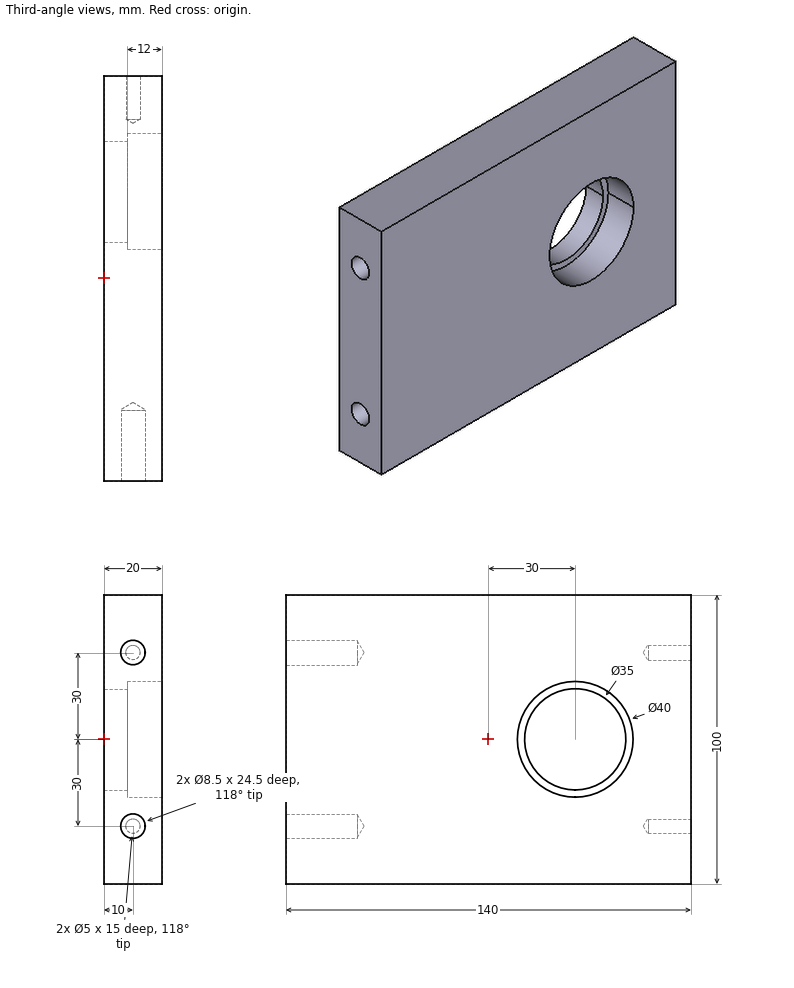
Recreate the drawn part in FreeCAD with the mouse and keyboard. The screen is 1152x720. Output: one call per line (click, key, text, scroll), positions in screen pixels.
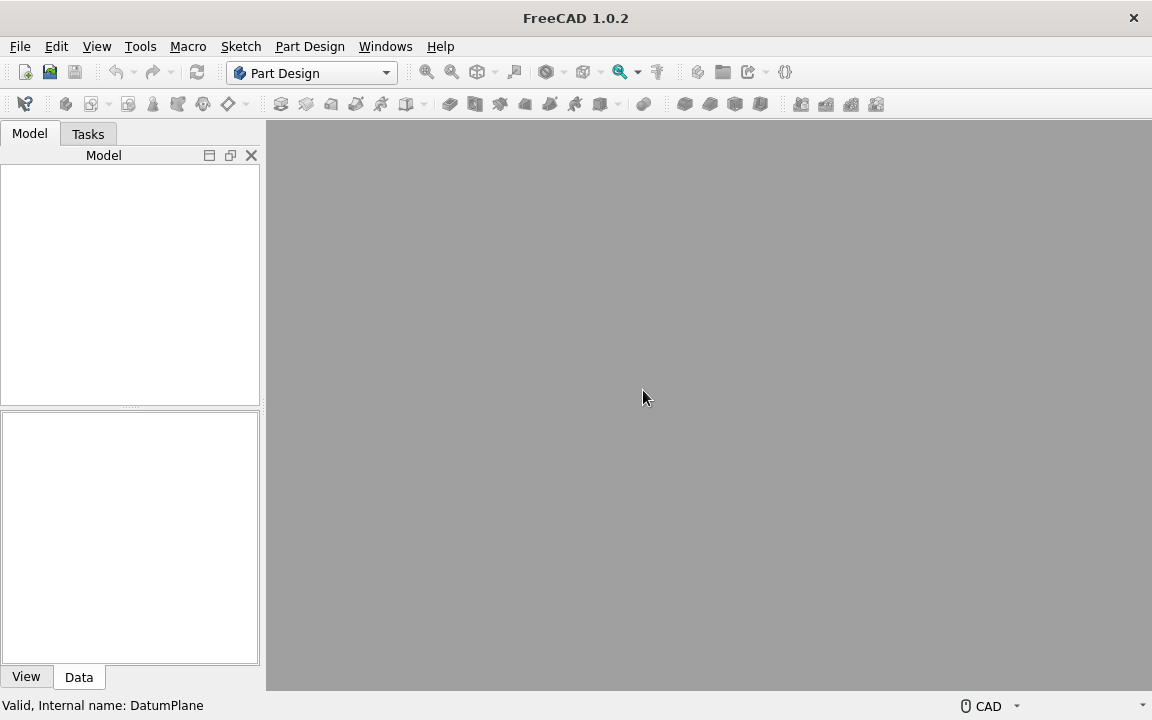
key(ctrl+n)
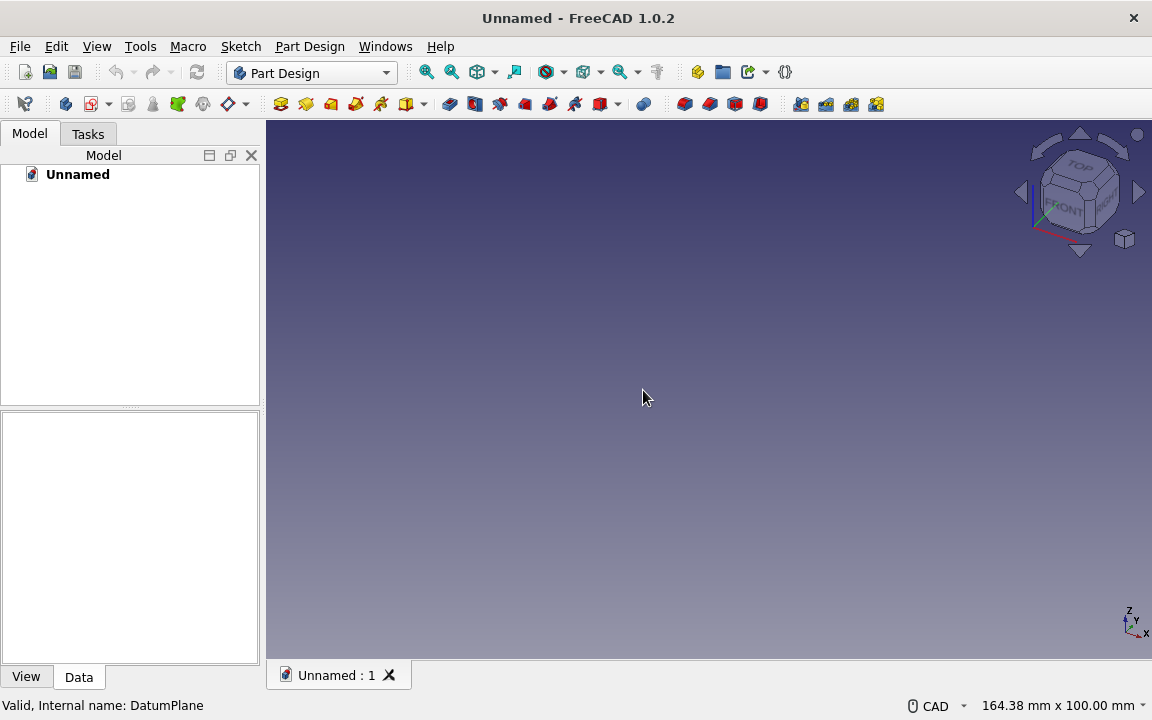
click(90, 104)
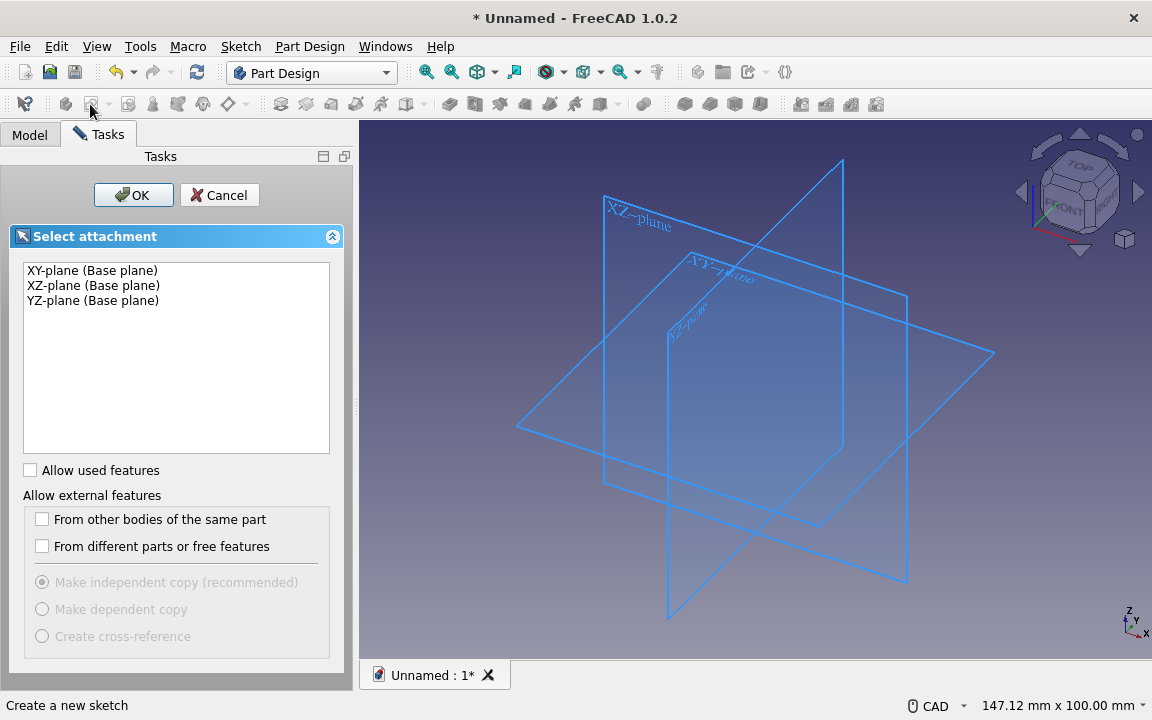
click(84, 300)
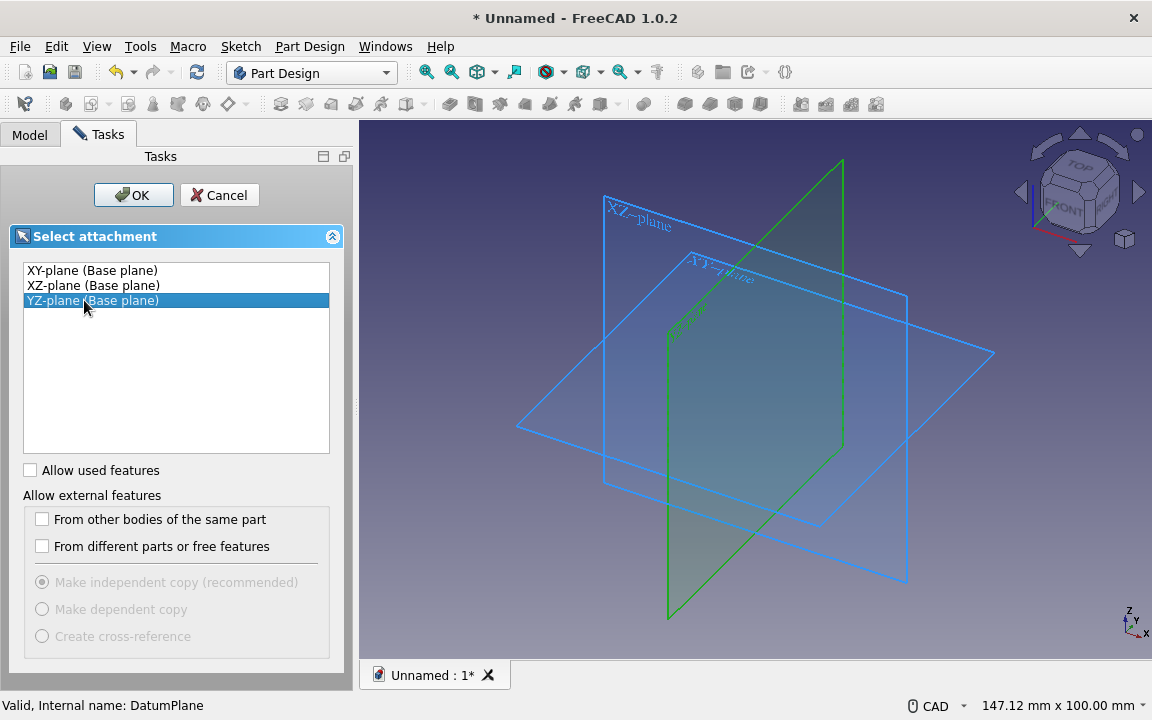
click(134, 195)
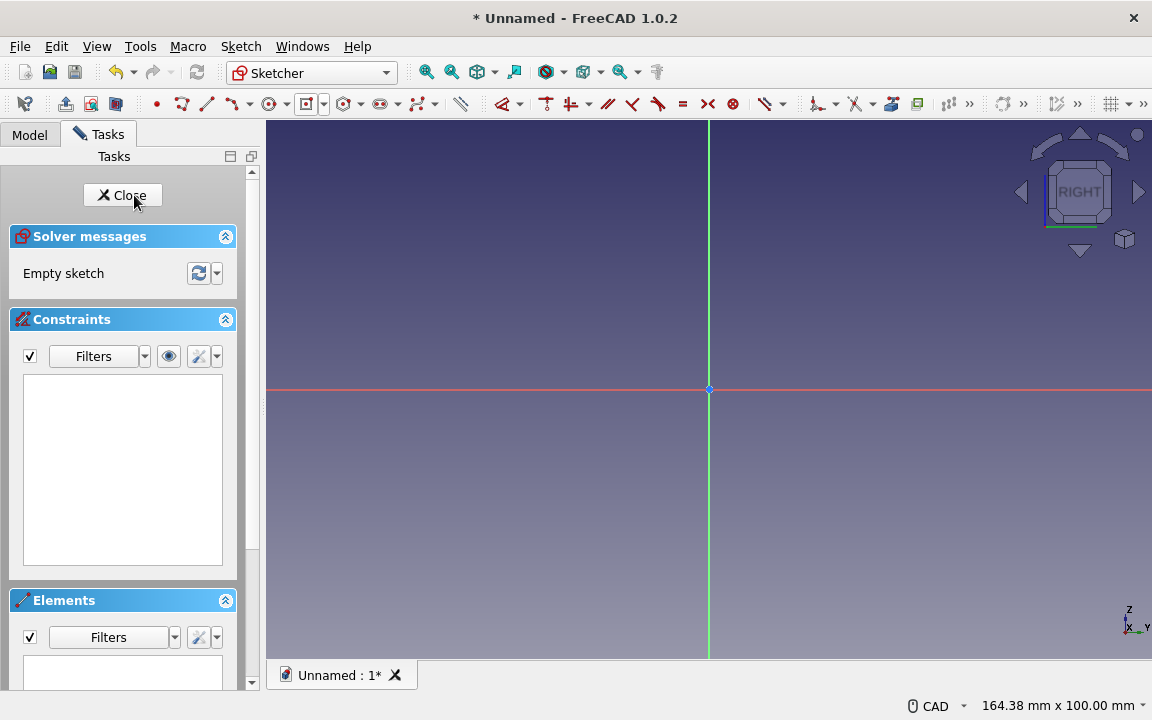
scroll(501, 390, down, 2)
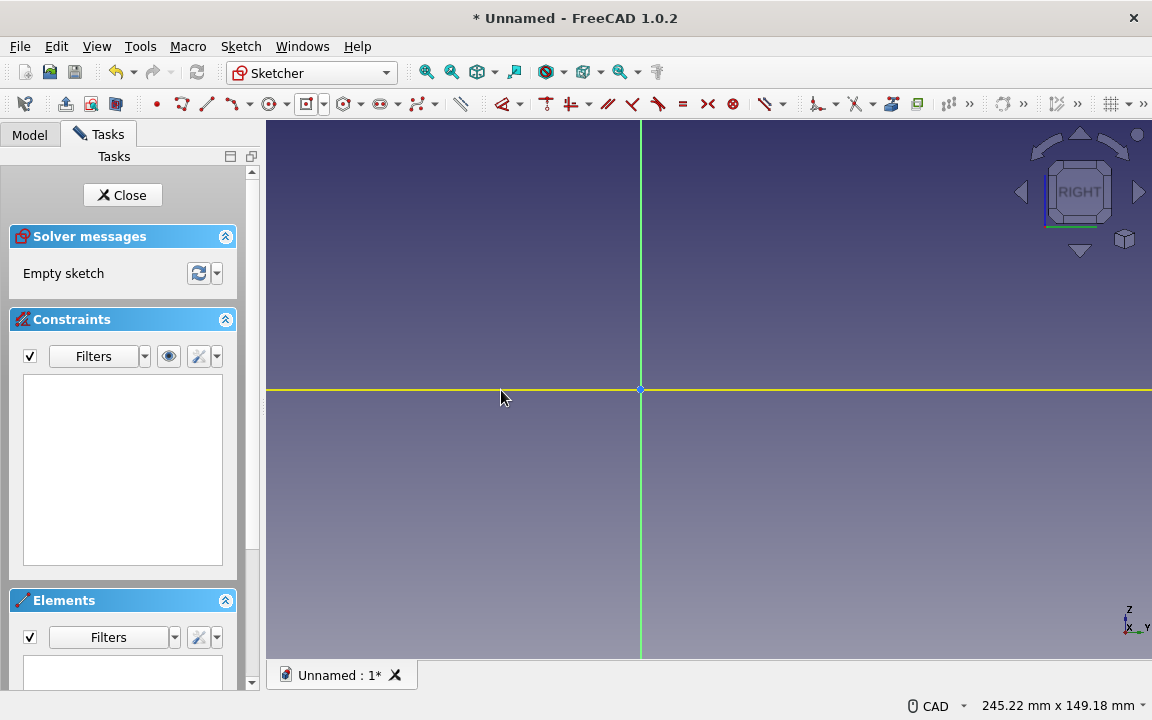
click(306, 104)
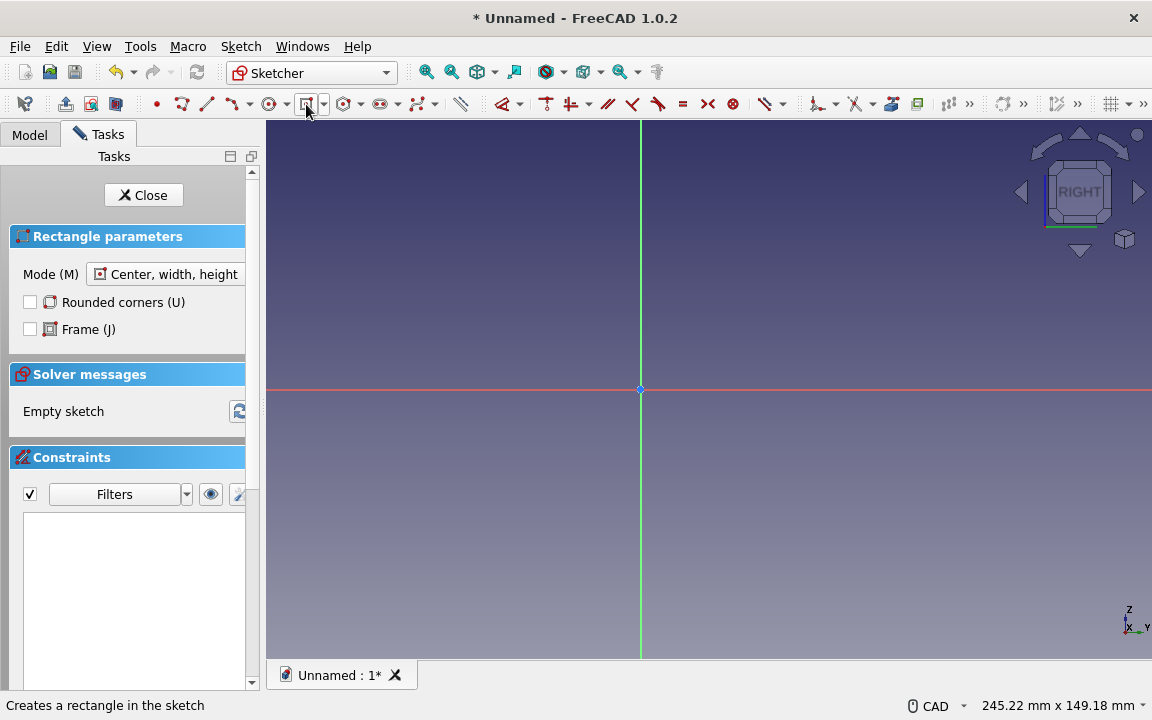
click(641, 390)
move(893, 209)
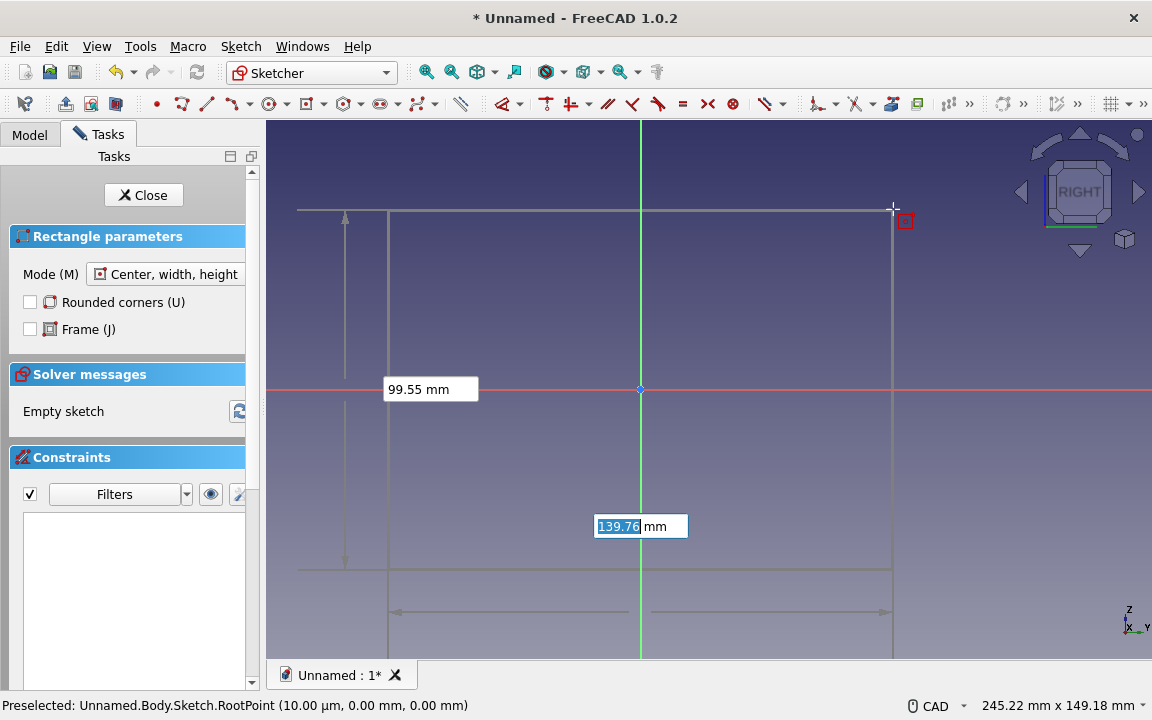
text(140)
key(Tab)
text(100)
key(Return)
key(Escape)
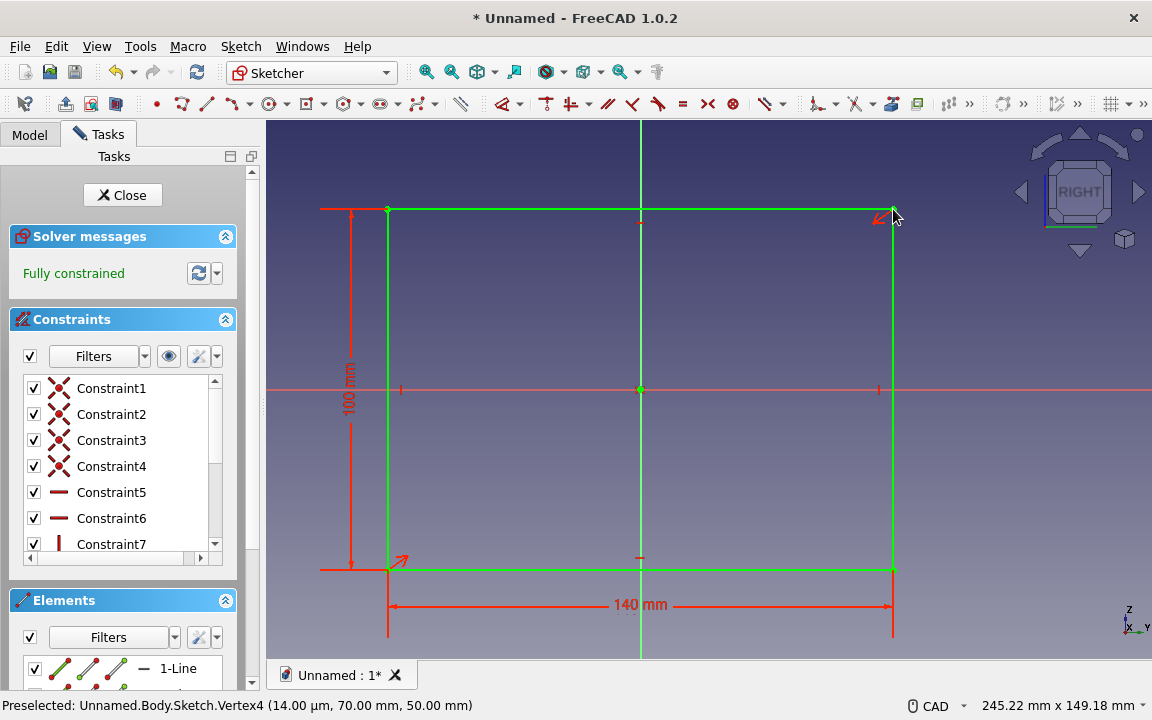
click(123, 195)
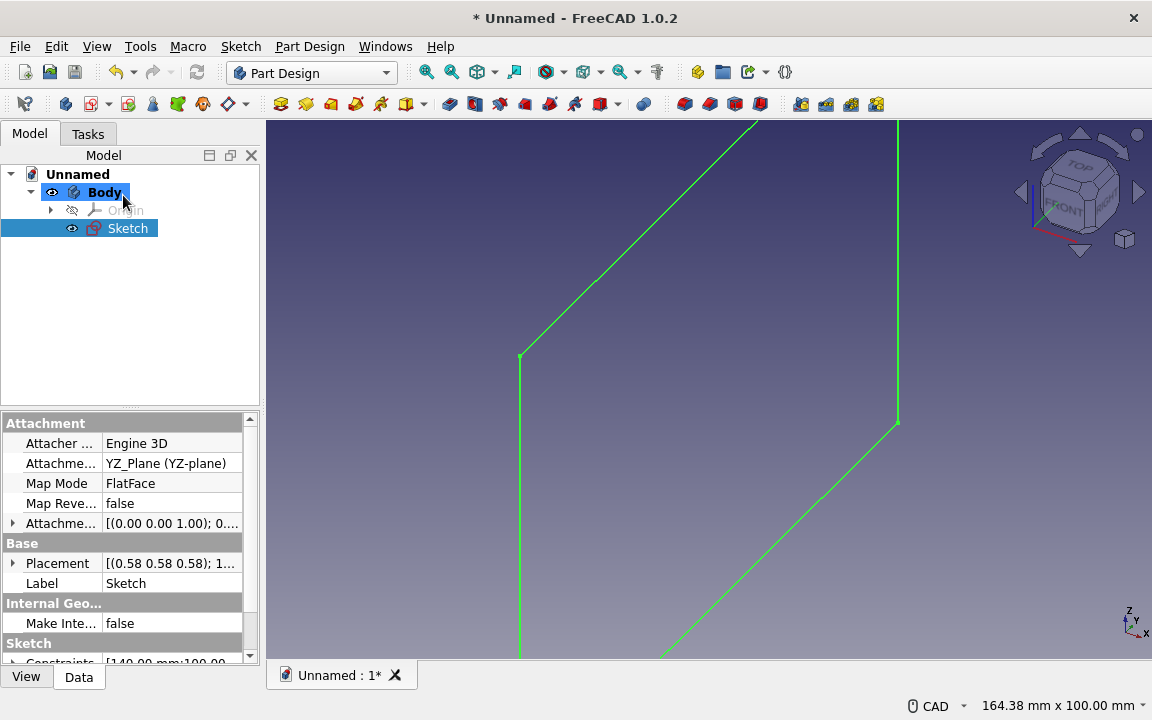
click(281, 104)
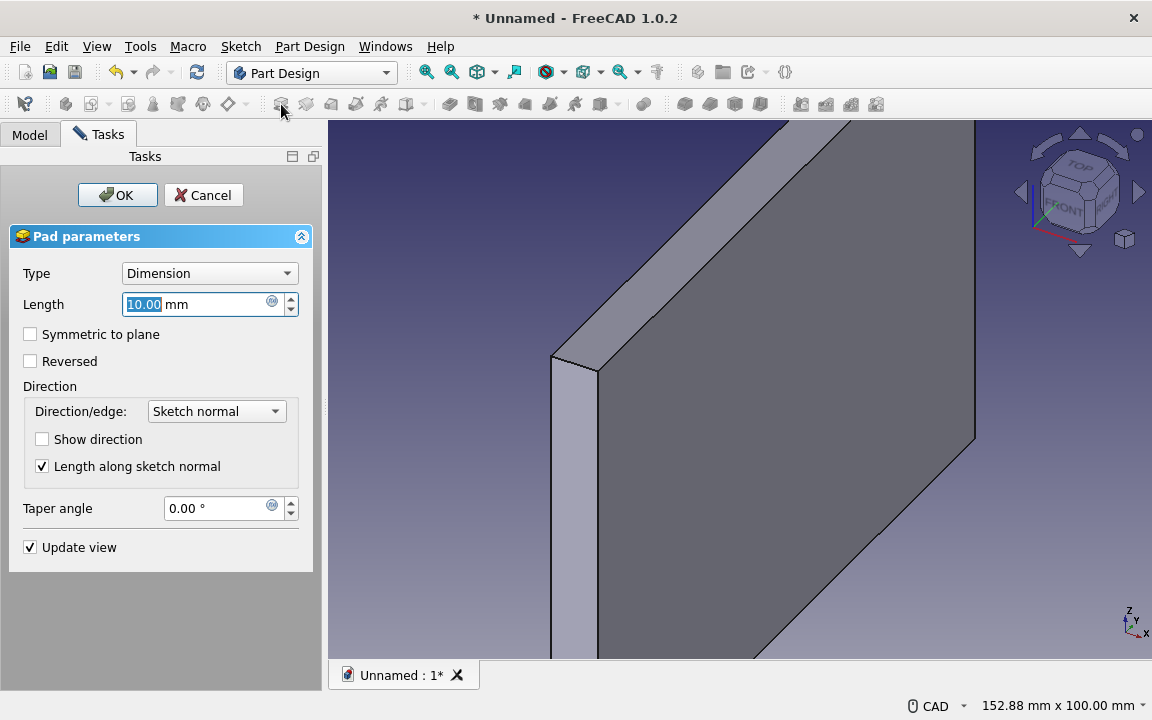
text(20)
key(Tab)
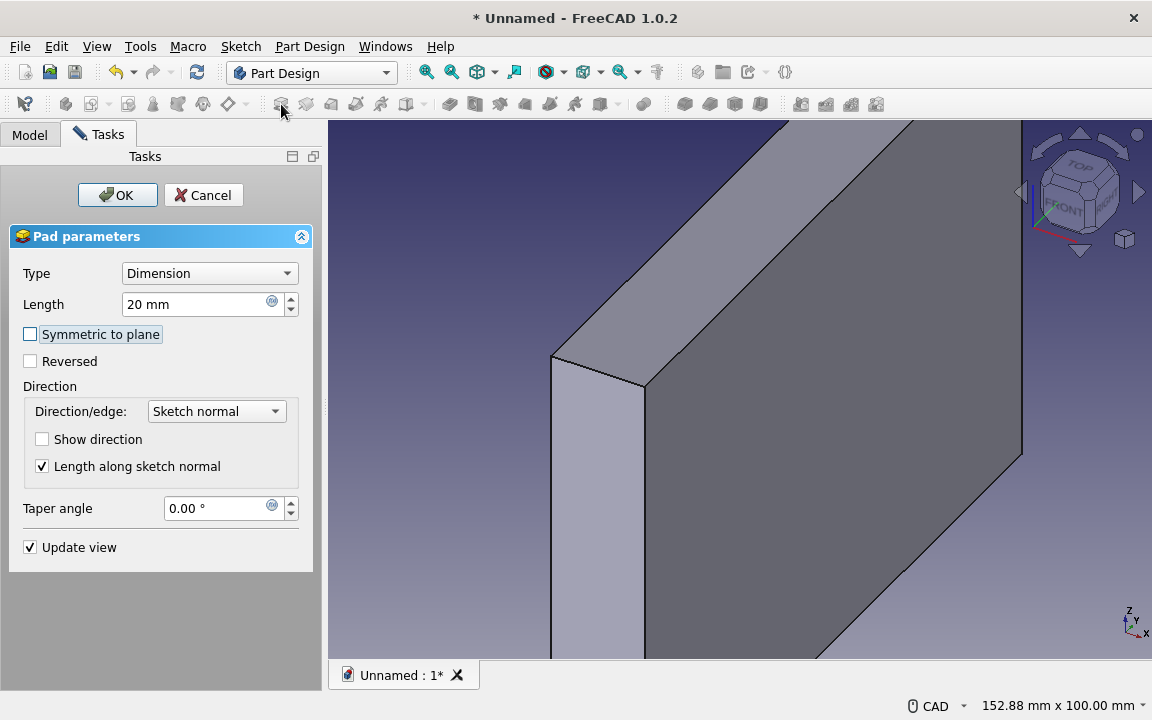
click(118, 195)